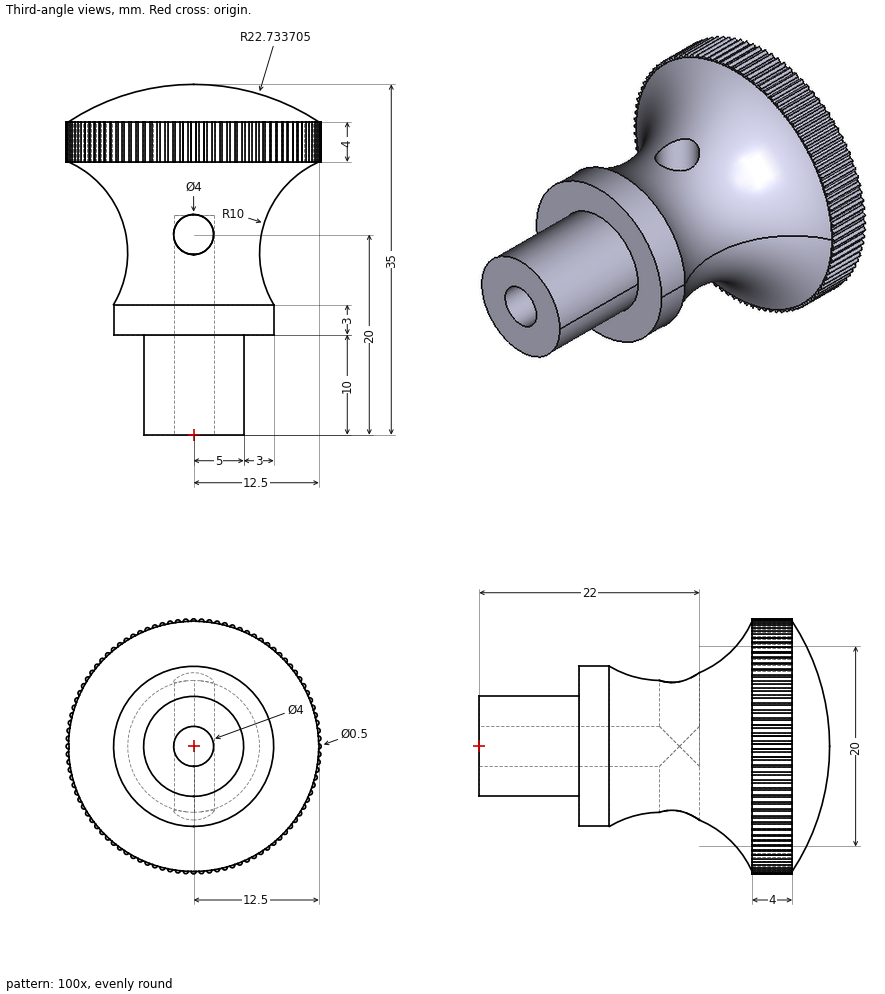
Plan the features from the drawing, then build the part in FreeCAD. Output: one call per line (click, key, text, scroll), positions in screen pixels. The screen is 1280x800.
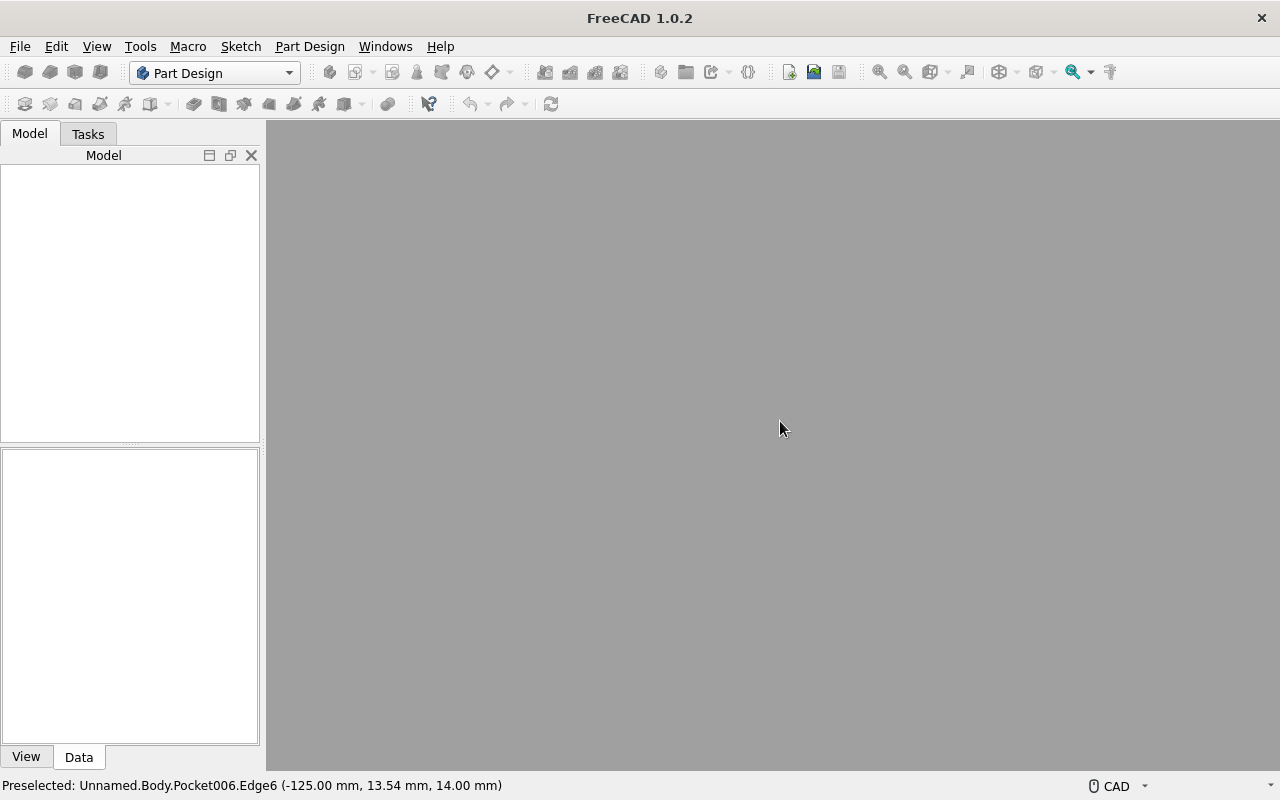
click(789, 72)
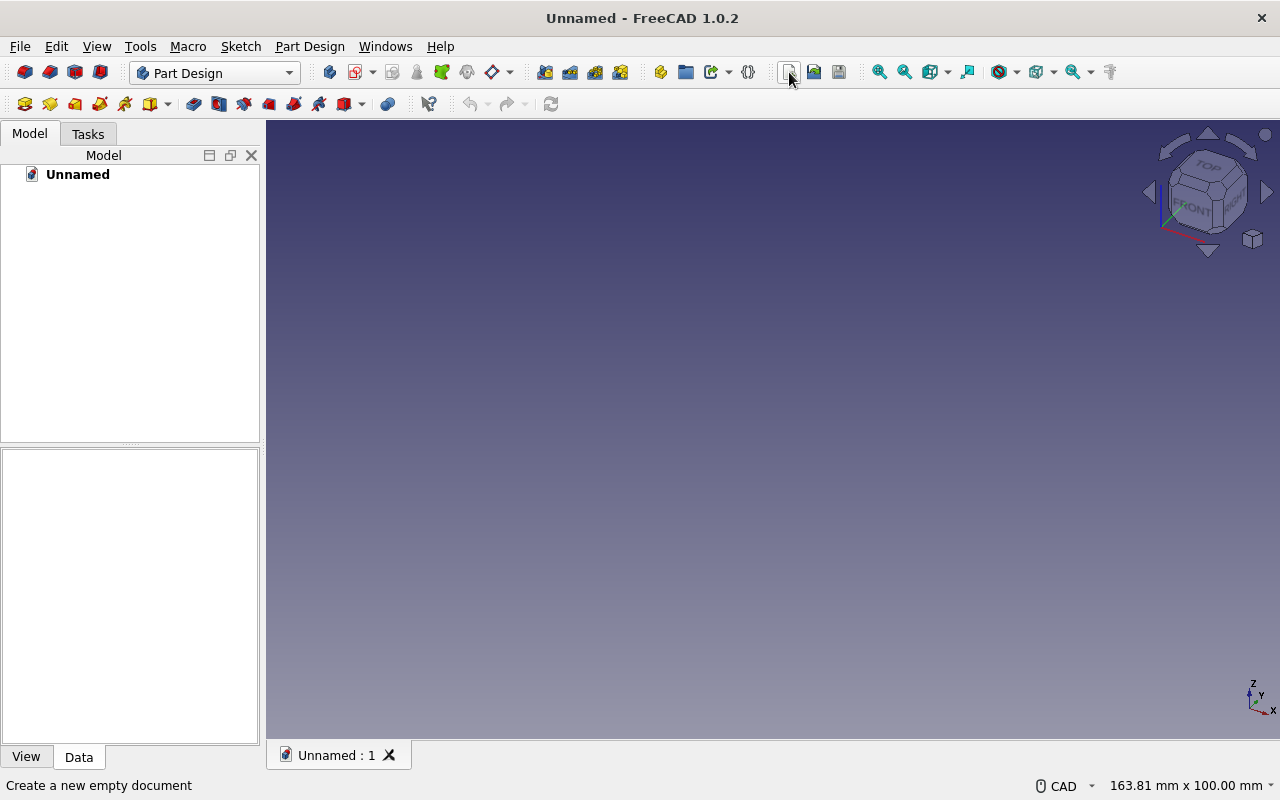
click(354, 72)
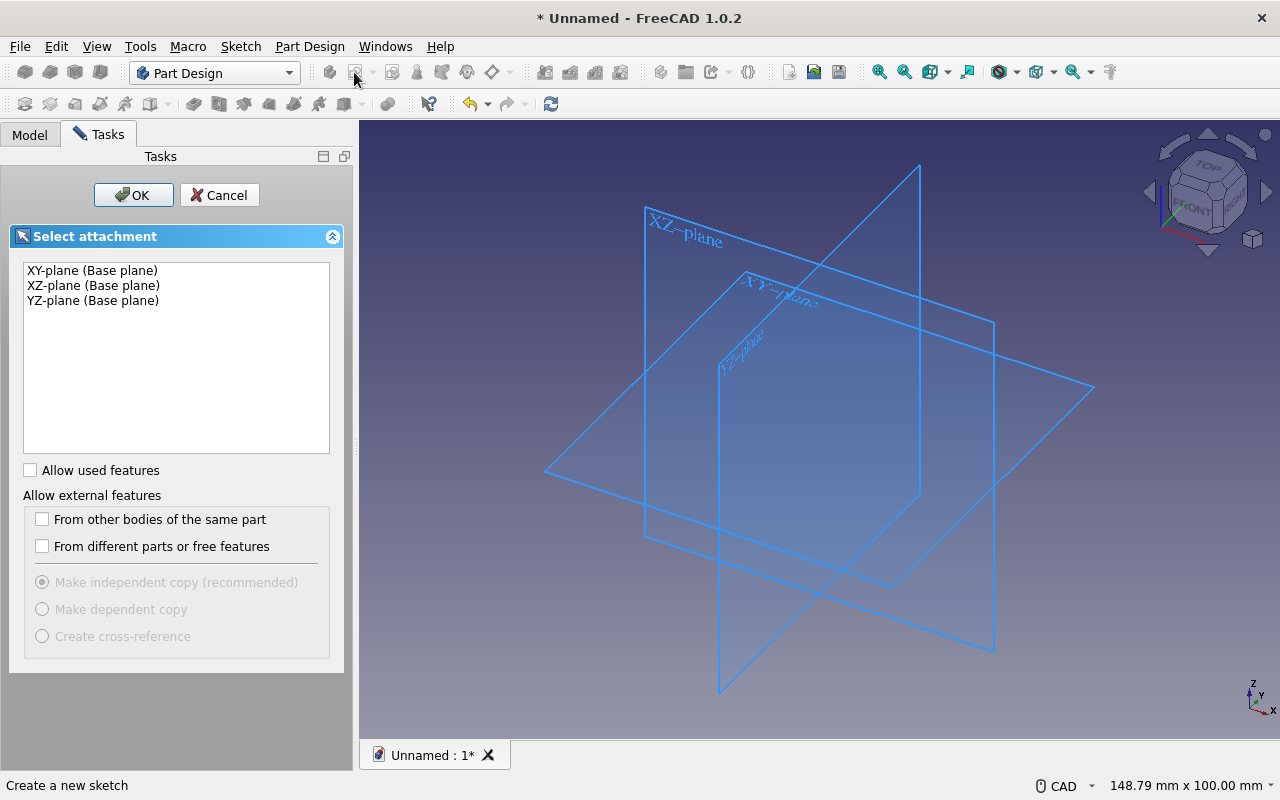
click(84, 270)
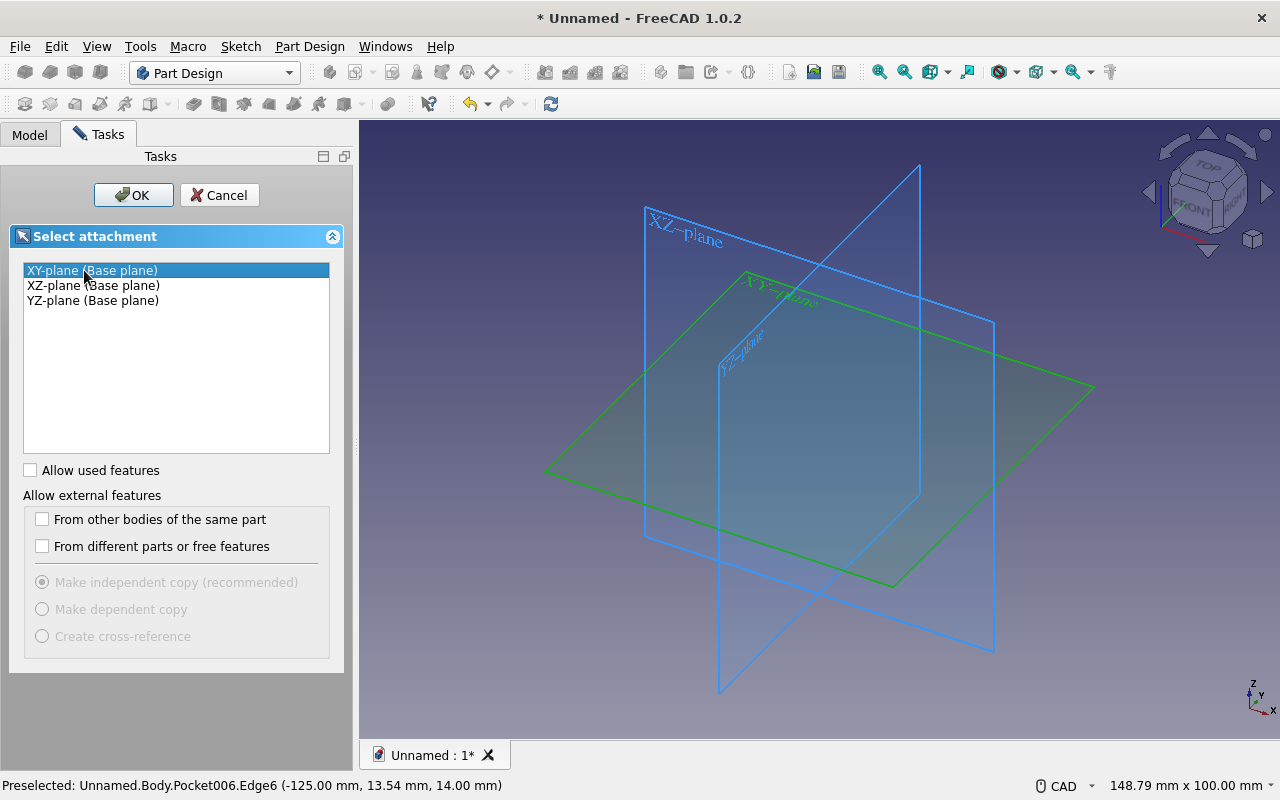
click(134, 195)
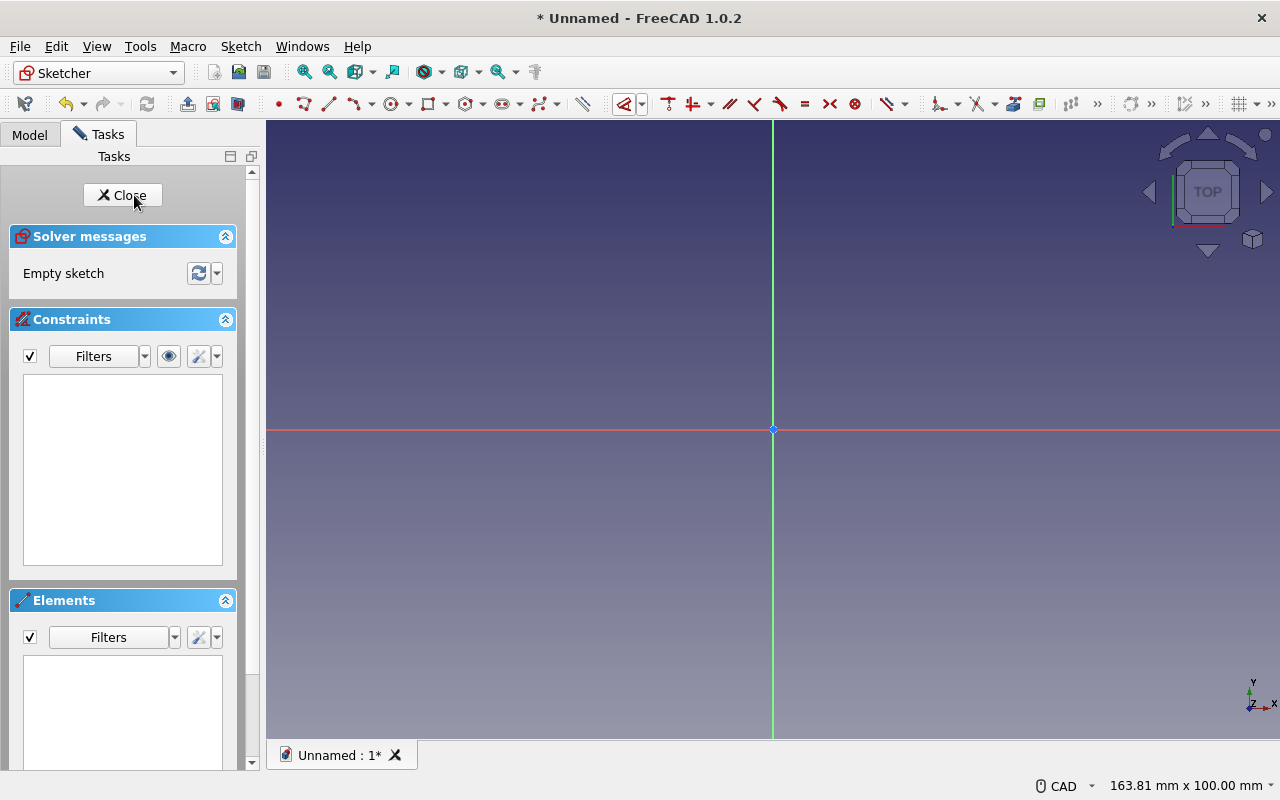
scroll(942, 189, up, 3)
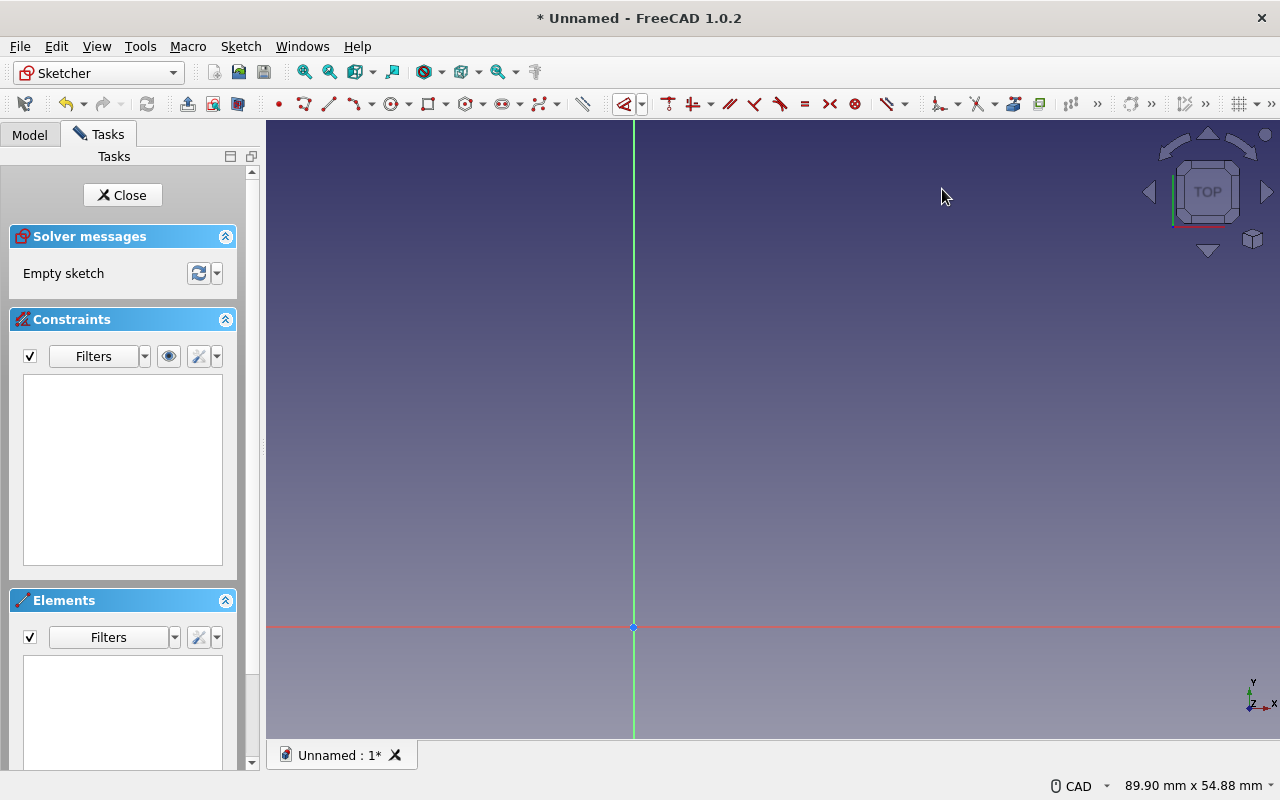
key(g)
key(m)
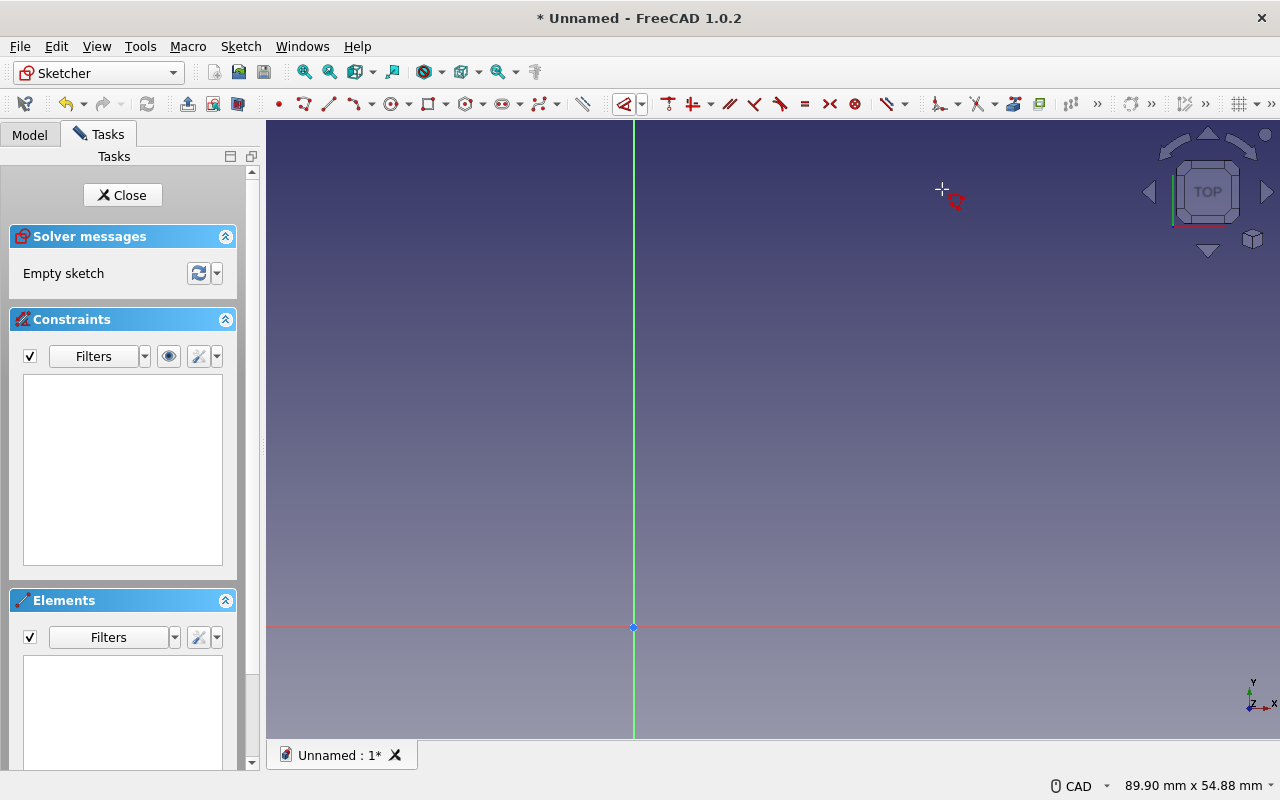
click(634, 232)
click(634, 627)
click(690, 618)
click(690, 514)
click(724, 514)
click(724, 481)
right_click(724, 481)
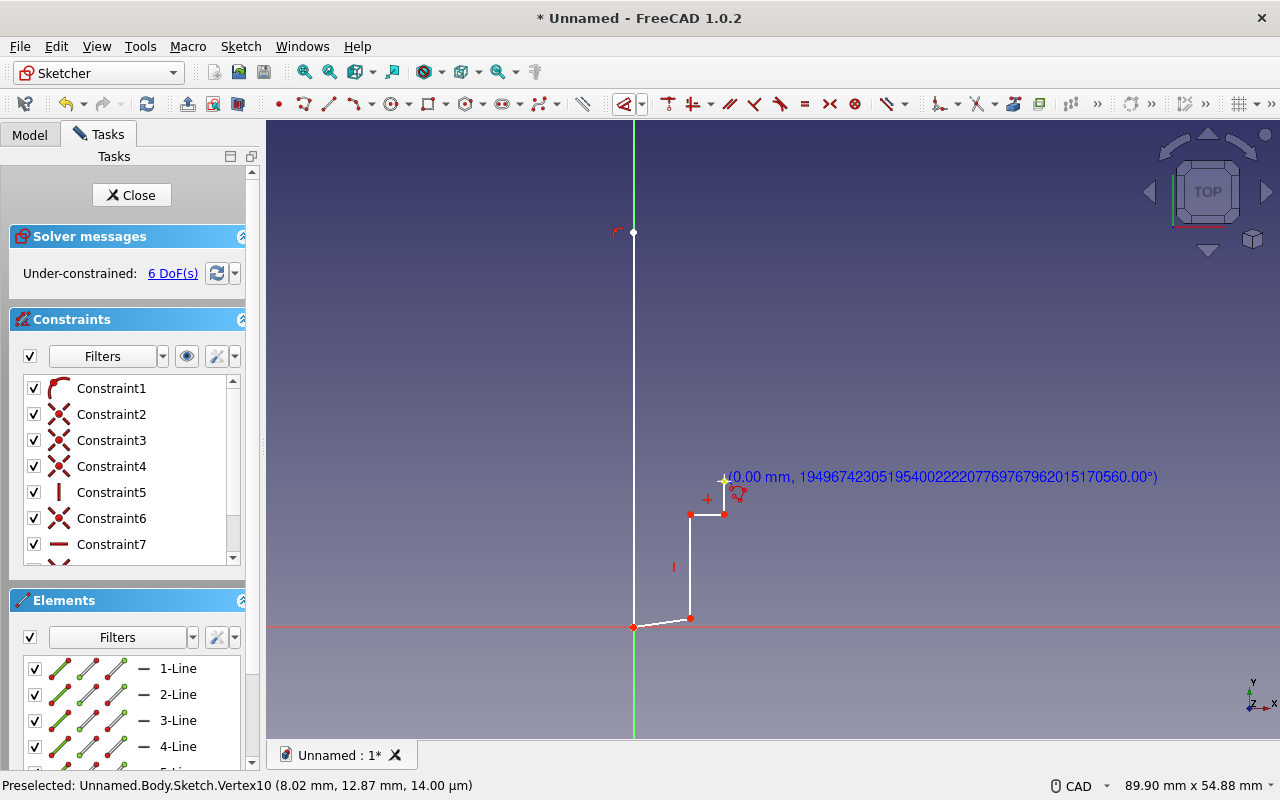
click(329, 104)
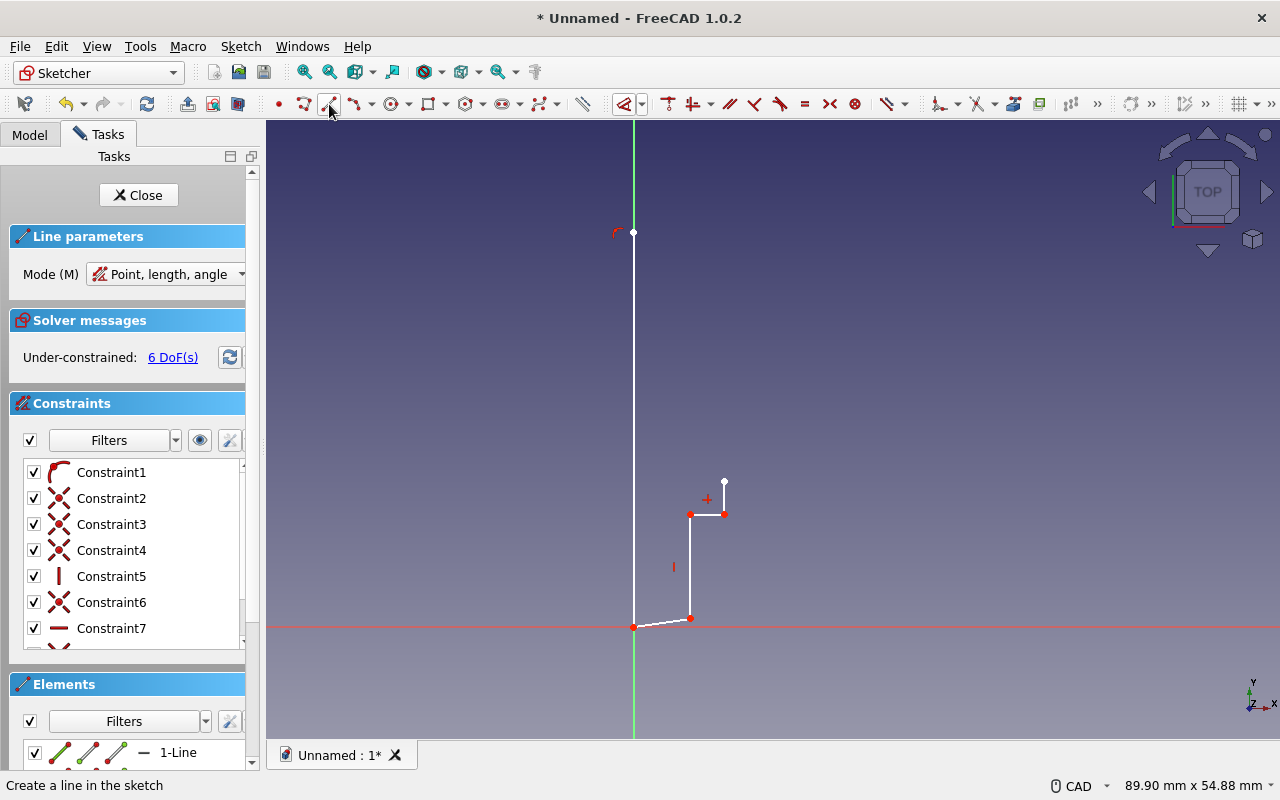
click(774, 320)
click(774, 275)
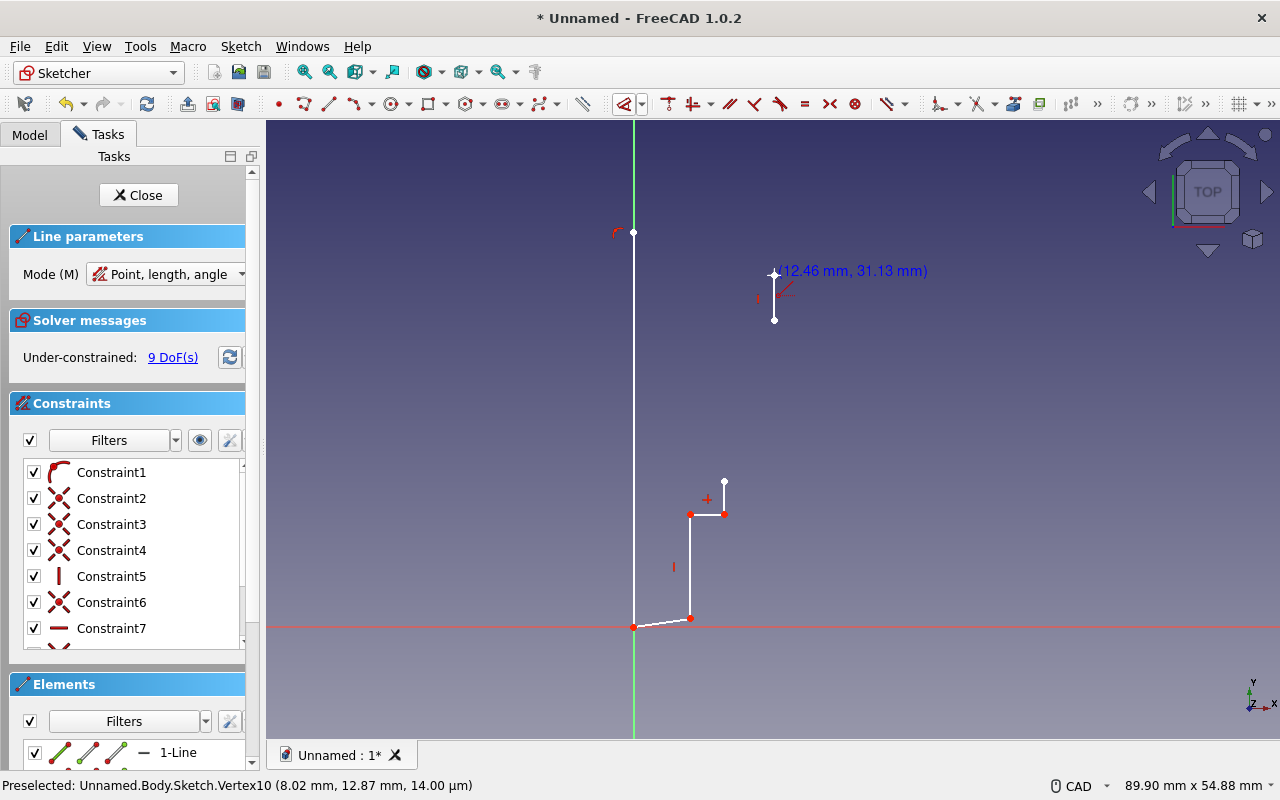
click(354, 104)